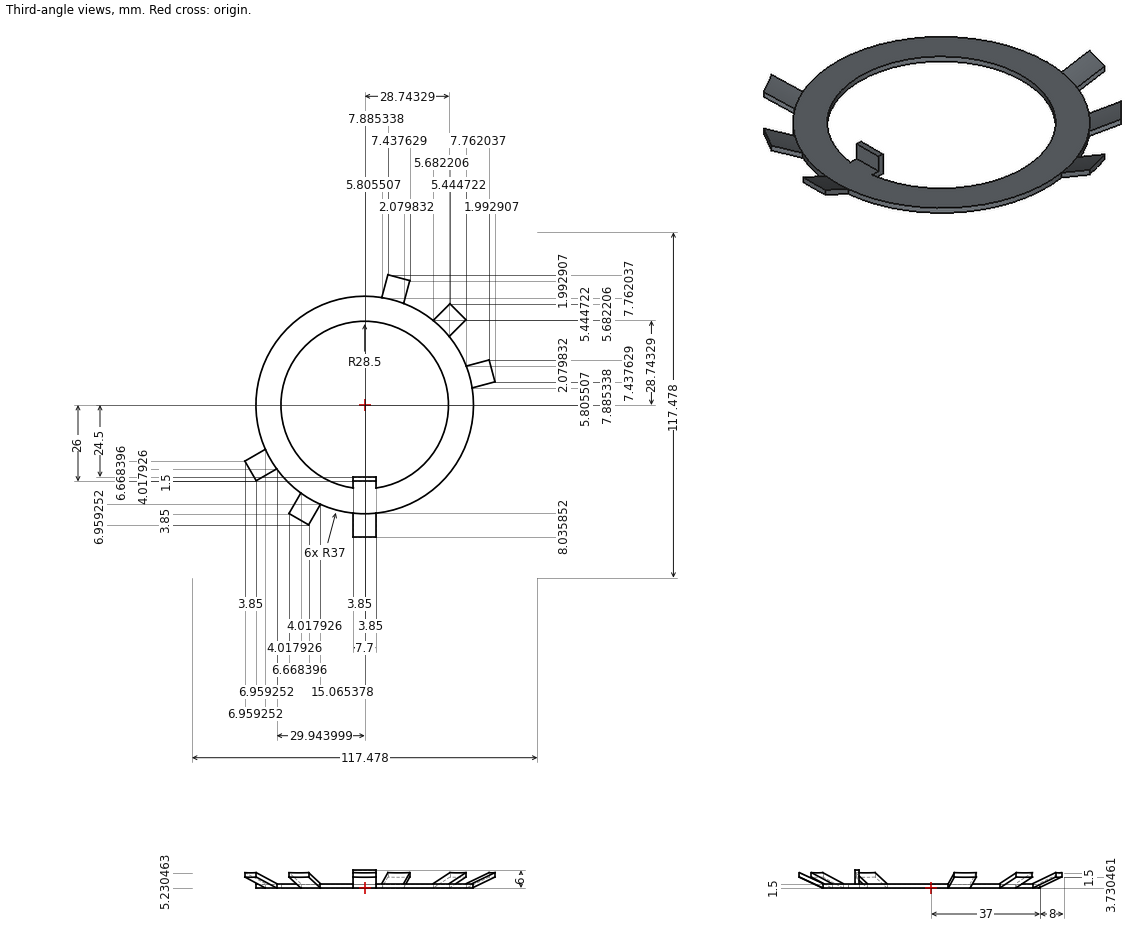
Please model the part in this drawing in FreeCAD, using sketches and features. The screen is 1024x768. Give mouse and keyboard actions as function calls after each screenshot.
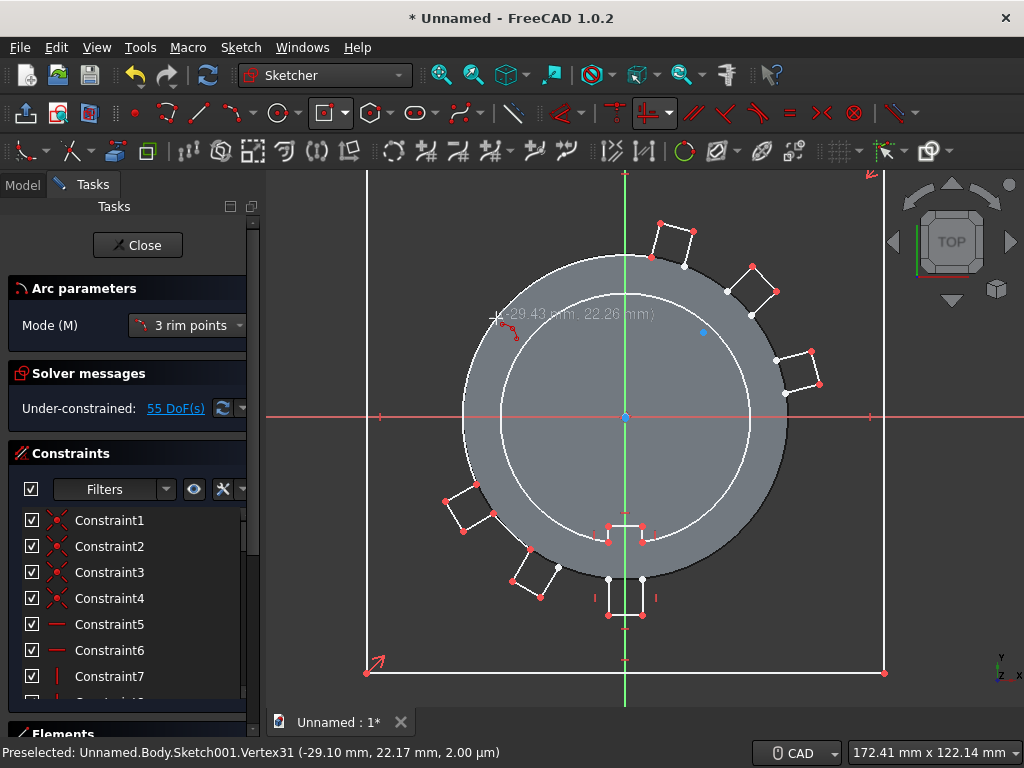
click(684, 266)
click(727, 292)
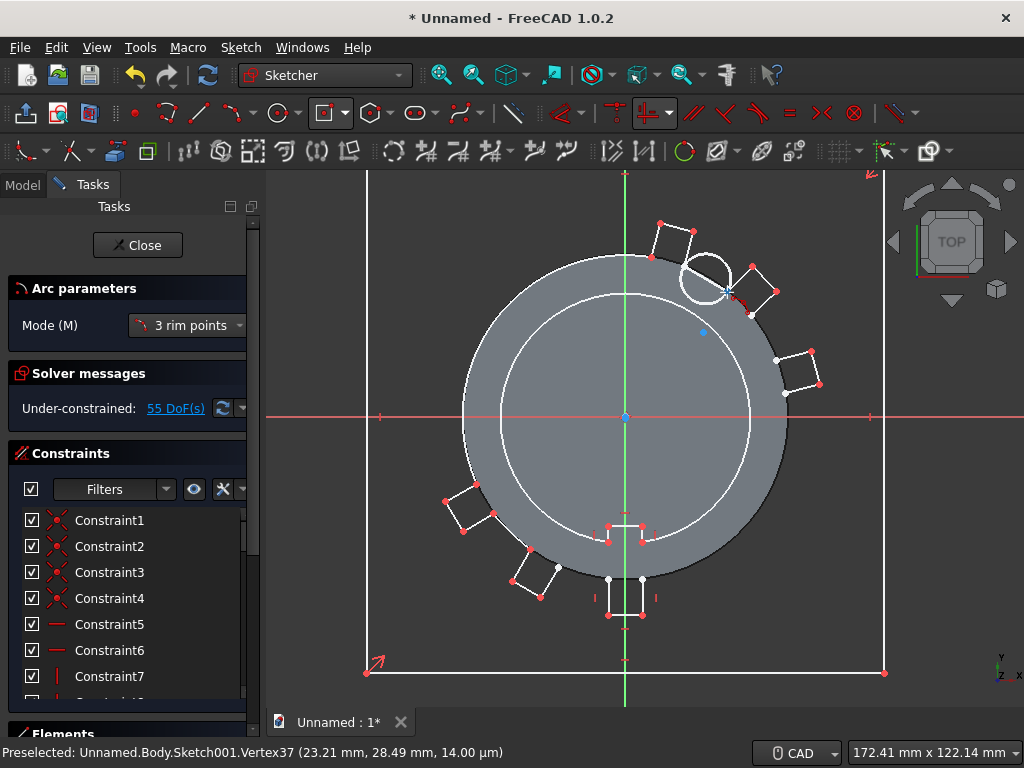
scroll(707, 276, up, 11)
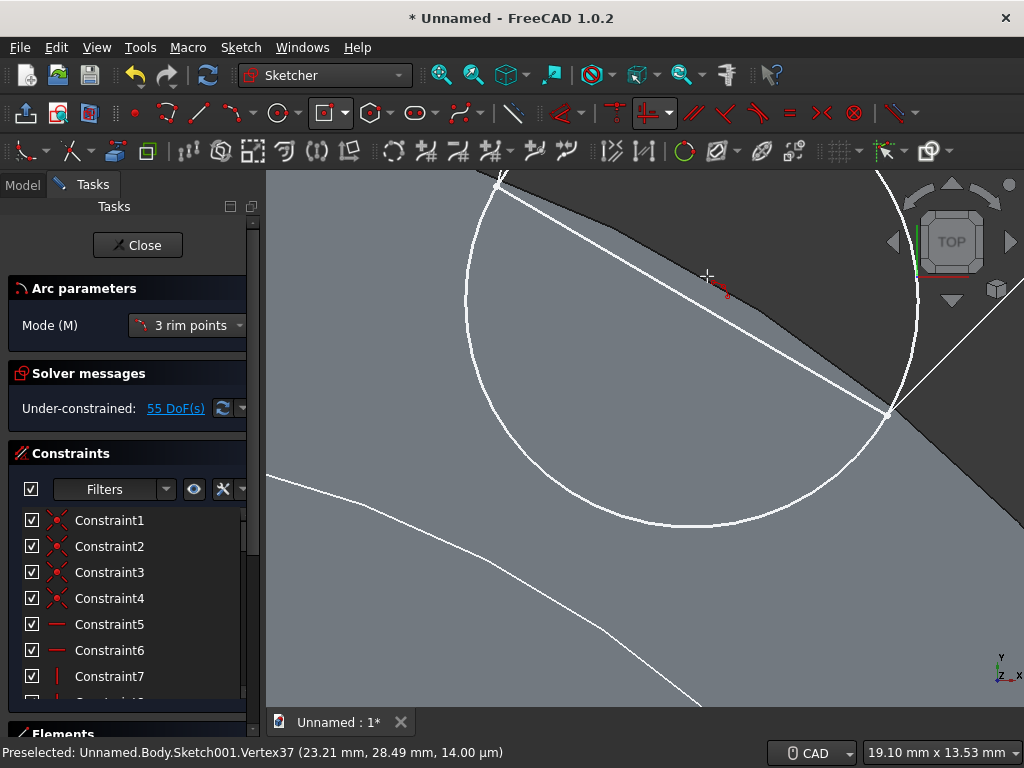
click(700, 274)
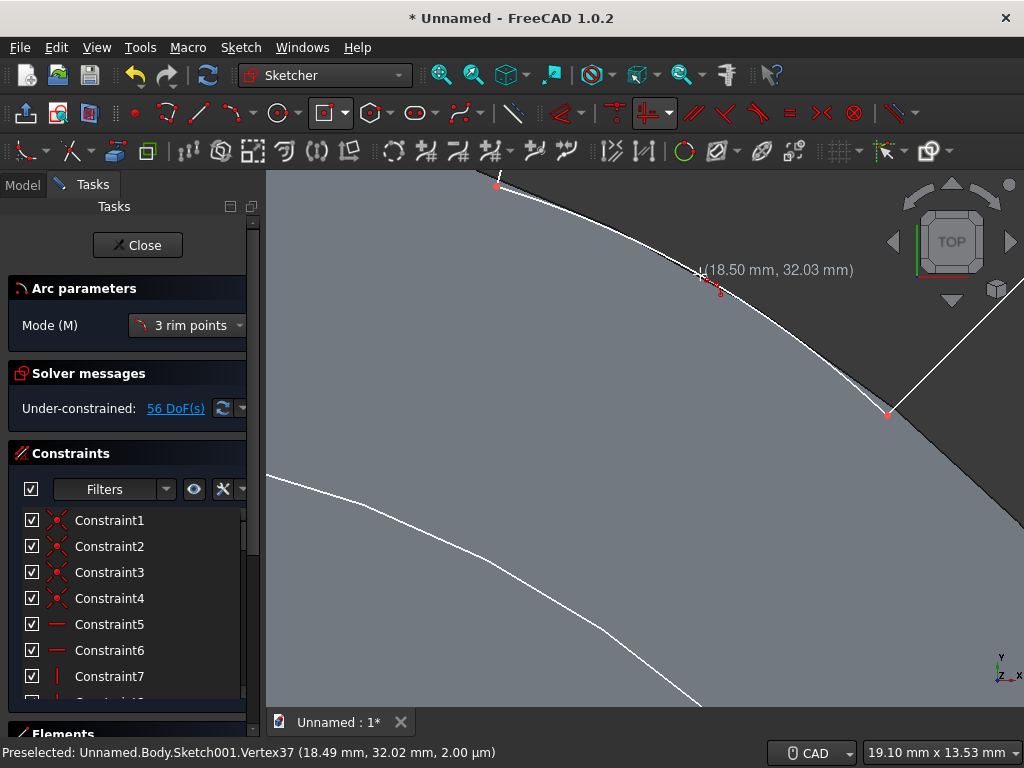
scroll(625, 350, down, 13)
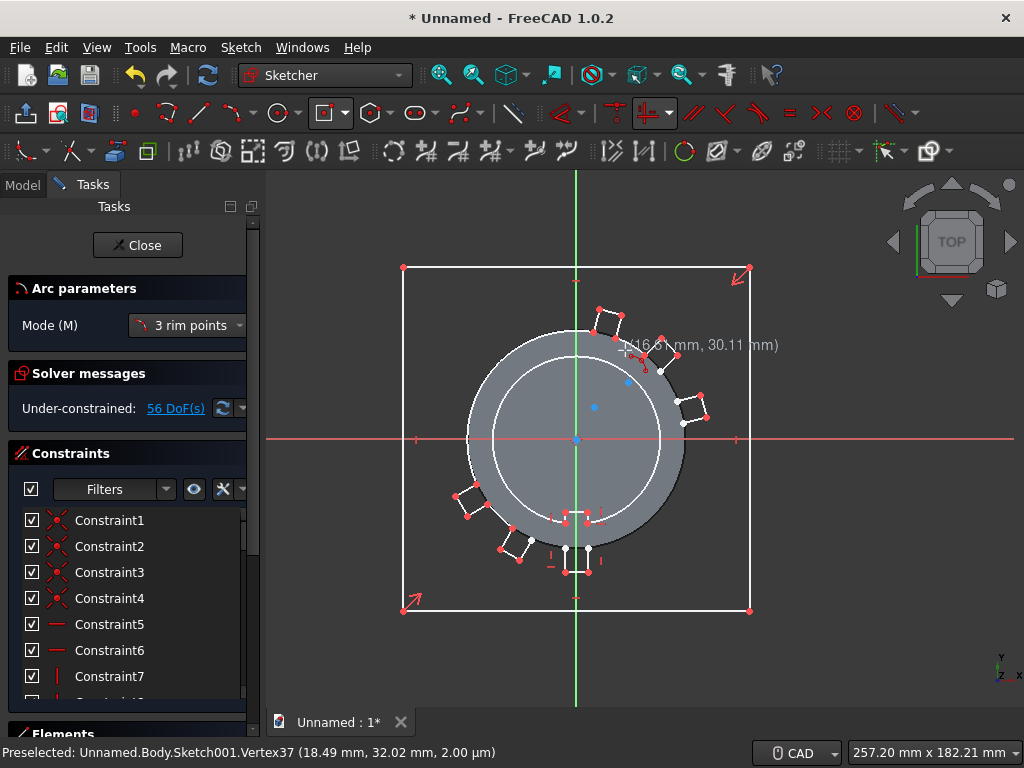
scroll(661, 370, up, 2)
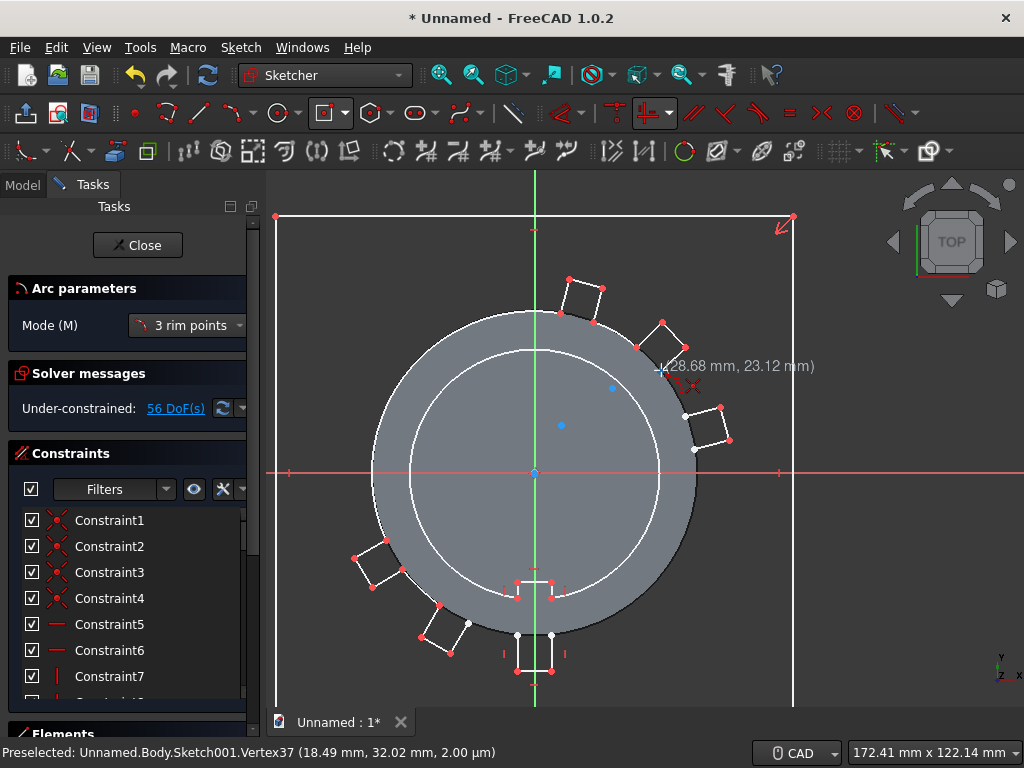
click(661, 372)
click(686, 416)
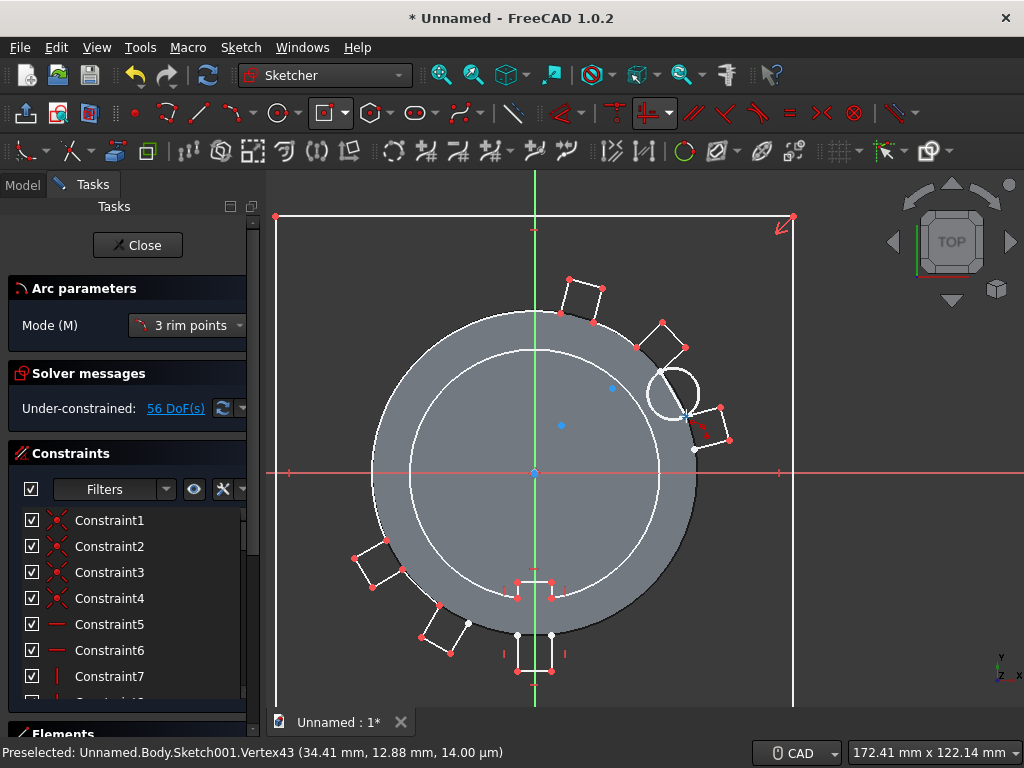
scroll(676, 392, up, 11)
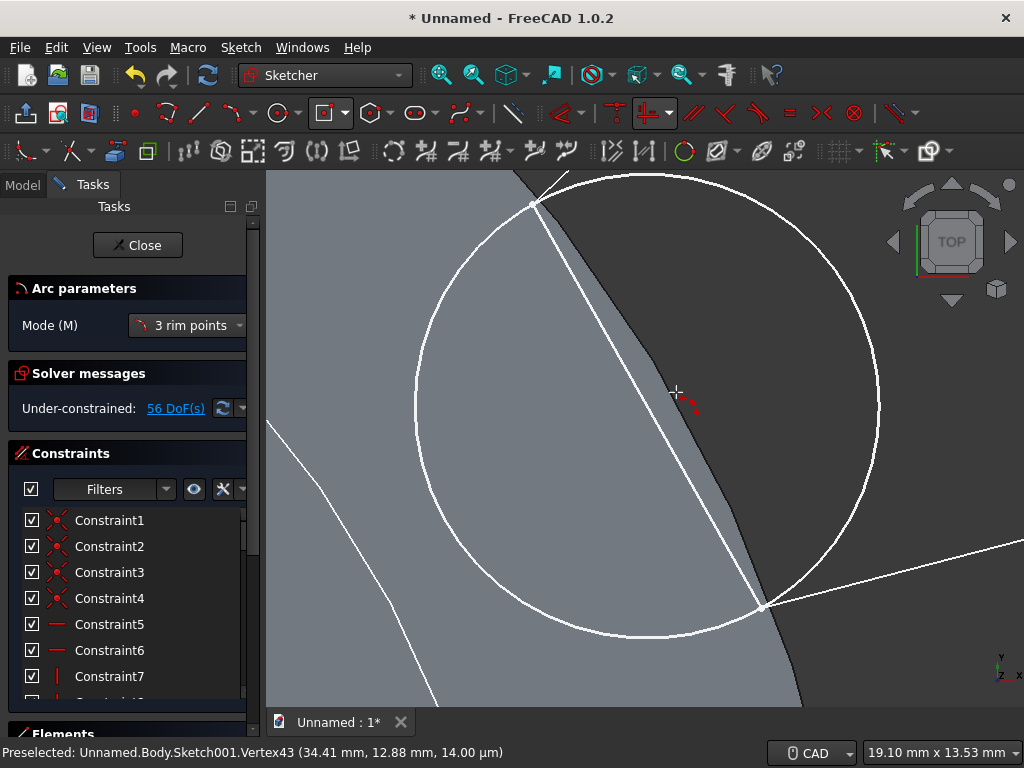
click(668, 385)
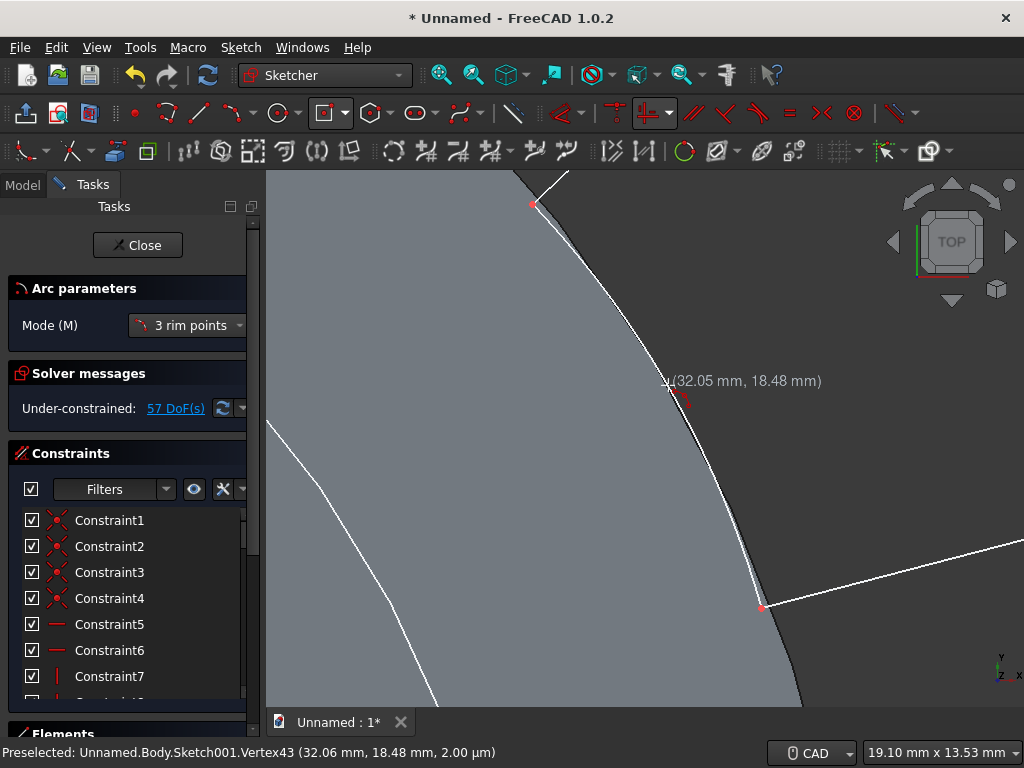
scroll(671, 384, down, 13)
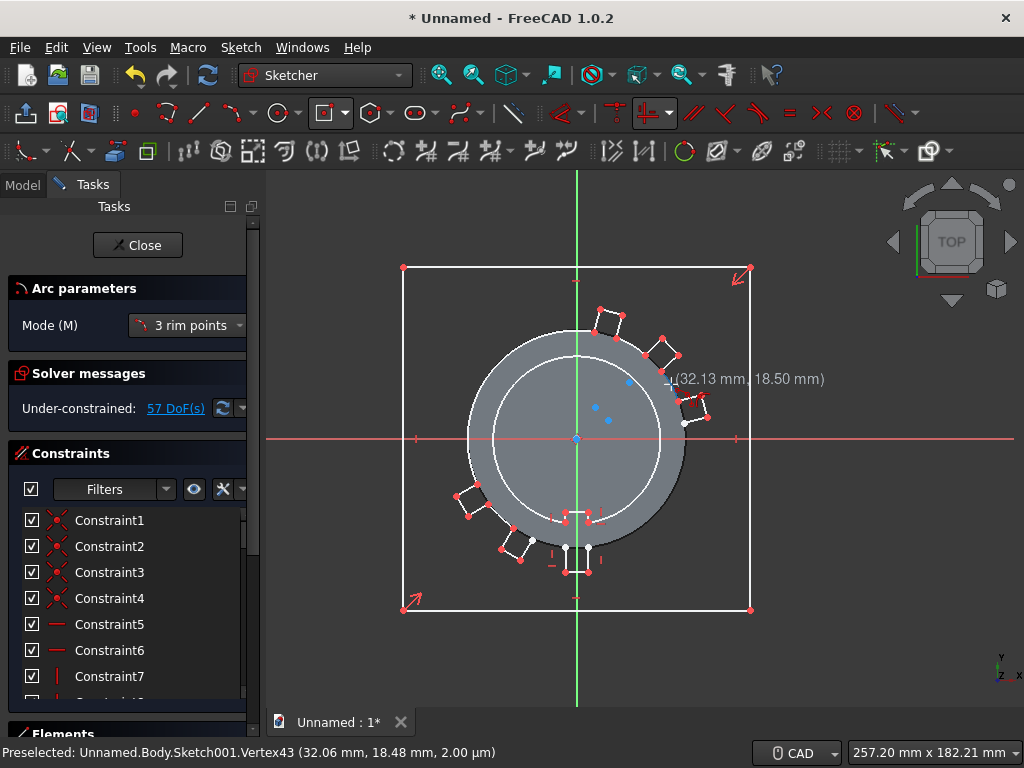
scroll(685, 422, up, 2)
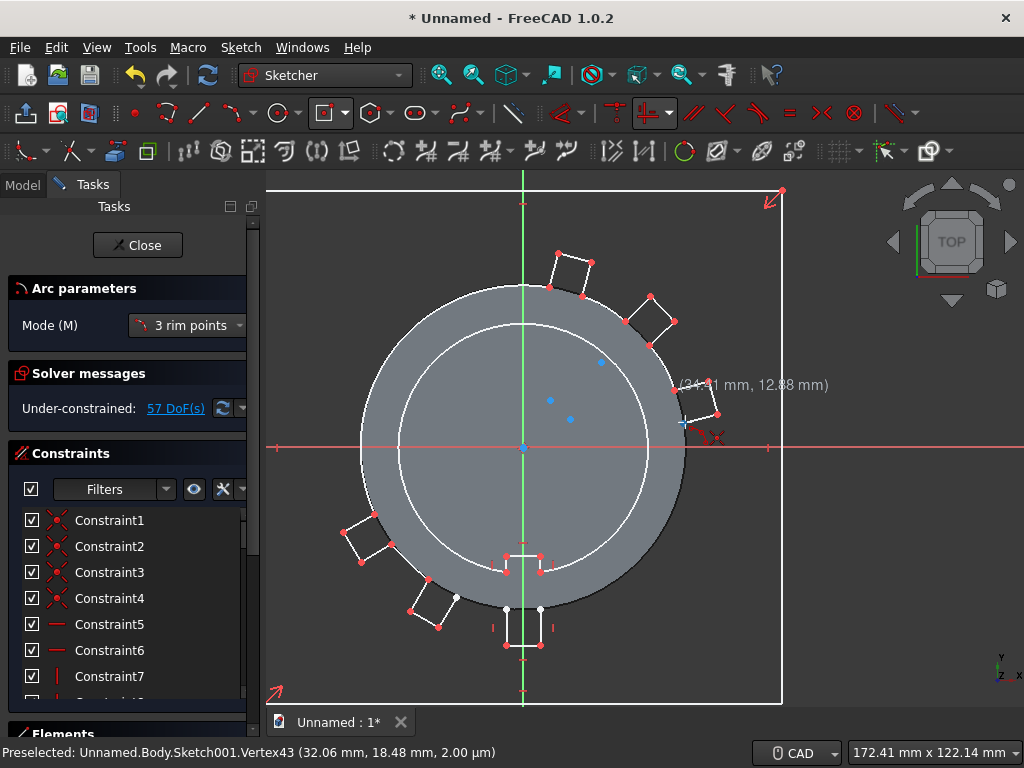
click(684, 423)
click(541, 610)
click(652, 546)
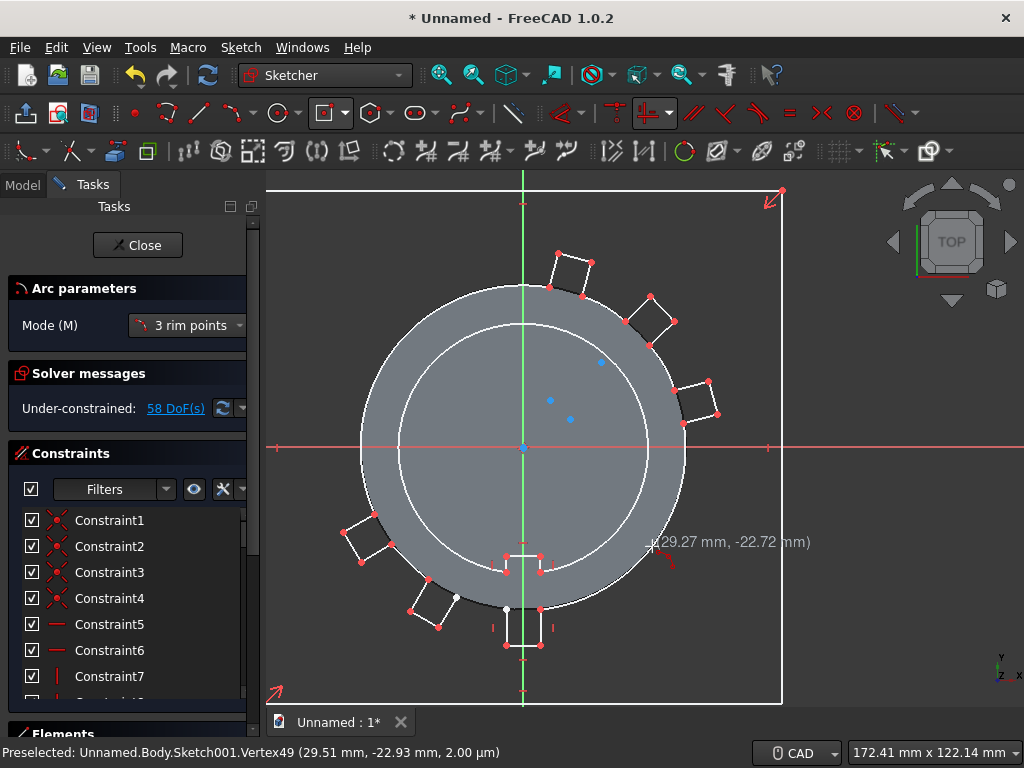
click(507, 610)
click(457, 598)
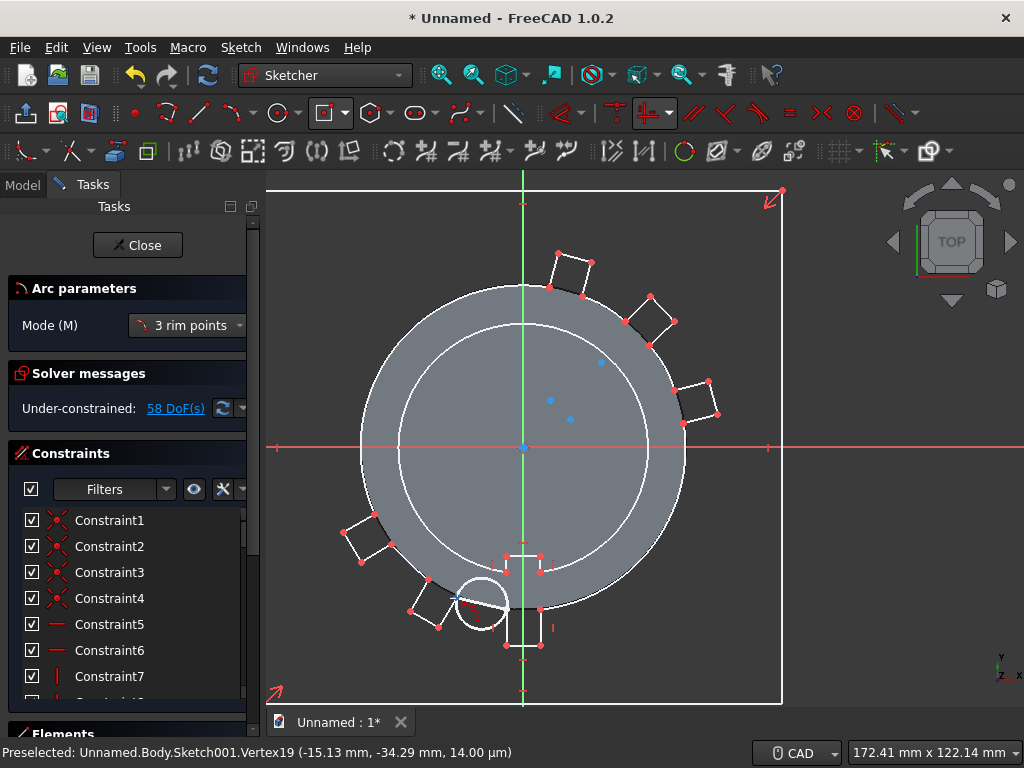
scroll(481, 604, up, 11)